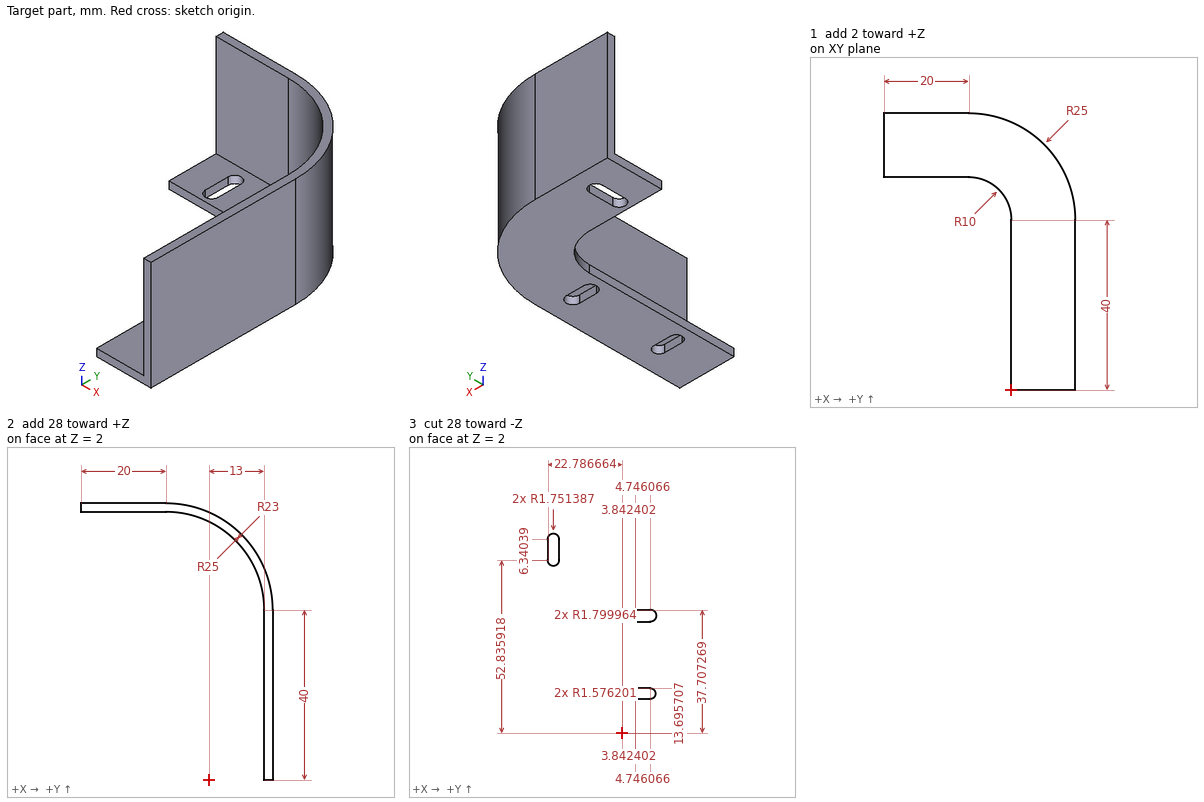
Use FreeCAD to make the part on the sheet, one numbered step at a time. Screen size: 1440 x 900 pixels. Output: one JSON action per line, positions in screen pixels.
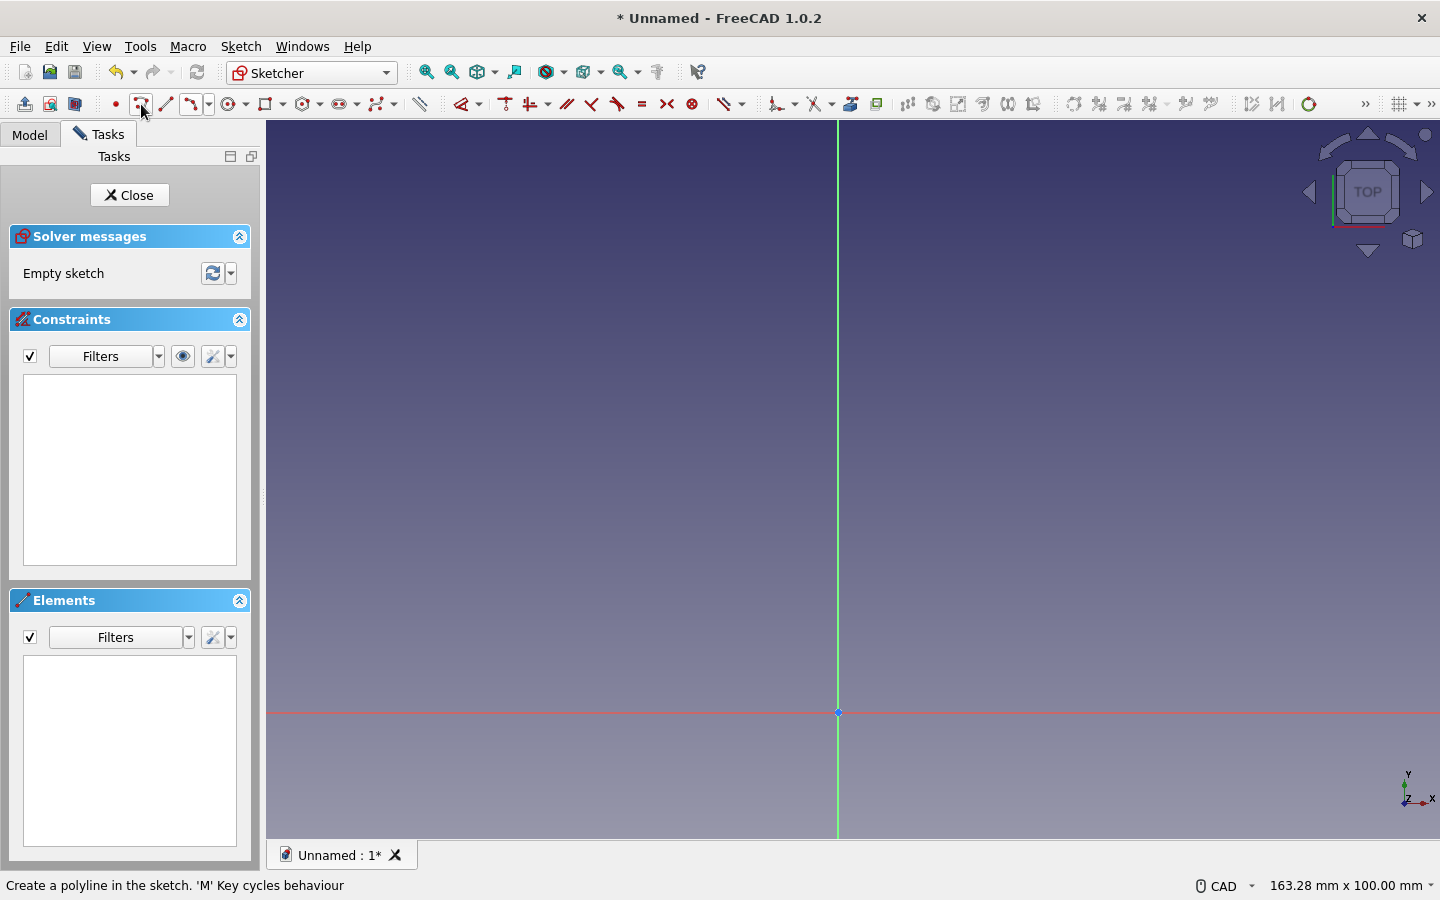
{"action": "left_click", "coordinate": [838, 425]}
{"action": "left_click", "coordinate": [838, 713]}
{"action": "left_click", "coordinate": [946, 704]}
{"action": "left_click", "coordinate": [946, 425]}
{"action": "right_click", "coordinate": [946, 425]}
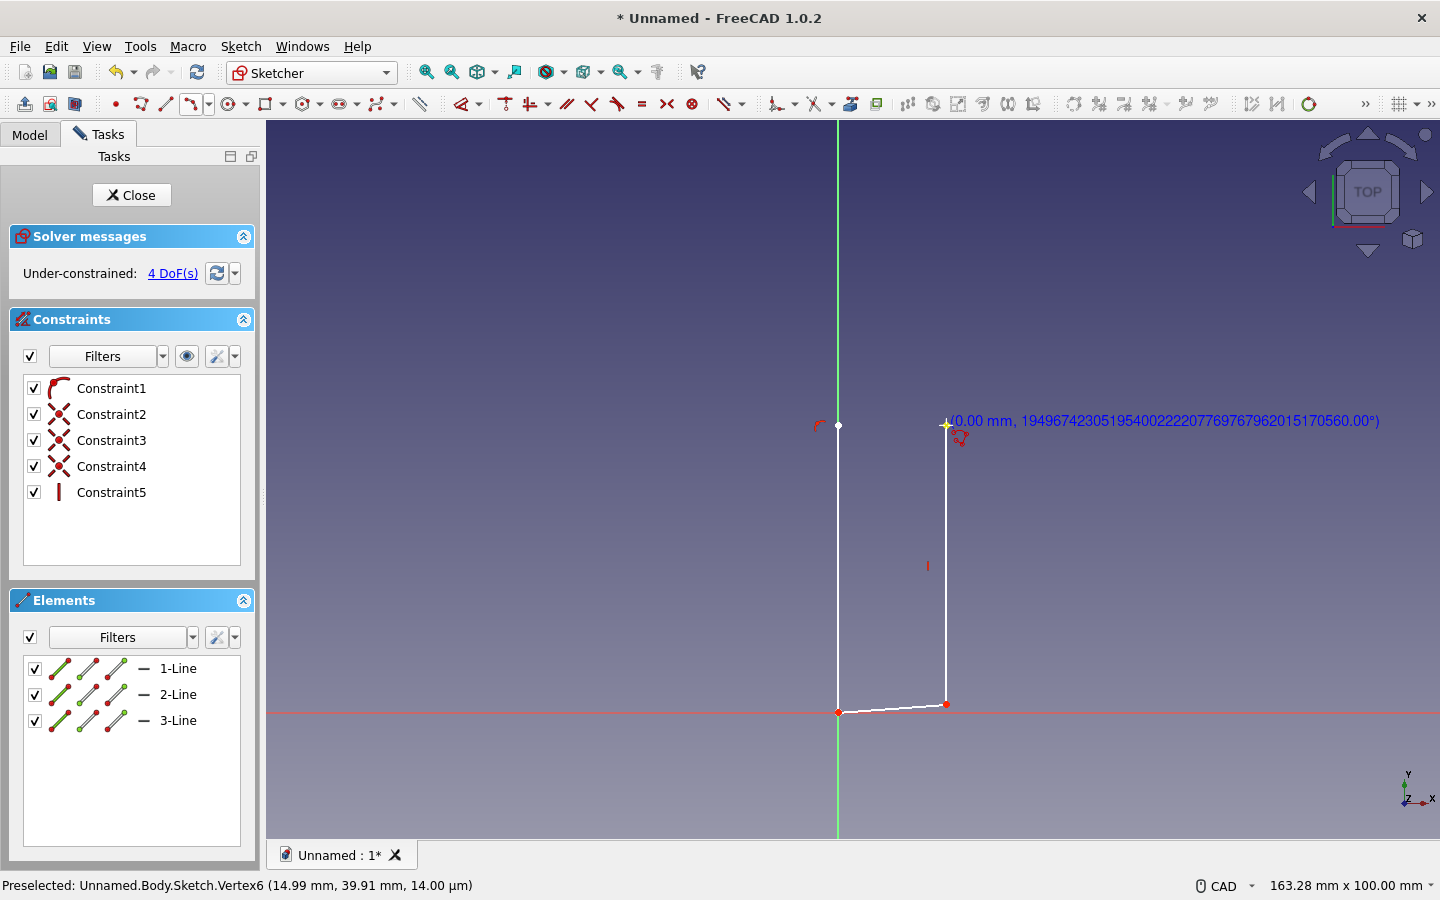
{"action": "left_click", "coordinate": [766, 246]}
{"action": "left_click", "coordinate": [623, 246]}
{"action": "left_click", "coordinate": [623, 353]}
{"action": "left_click", "coordinate": [766, 353]}
{"action": "right_click", "coordinate": [766, 353]}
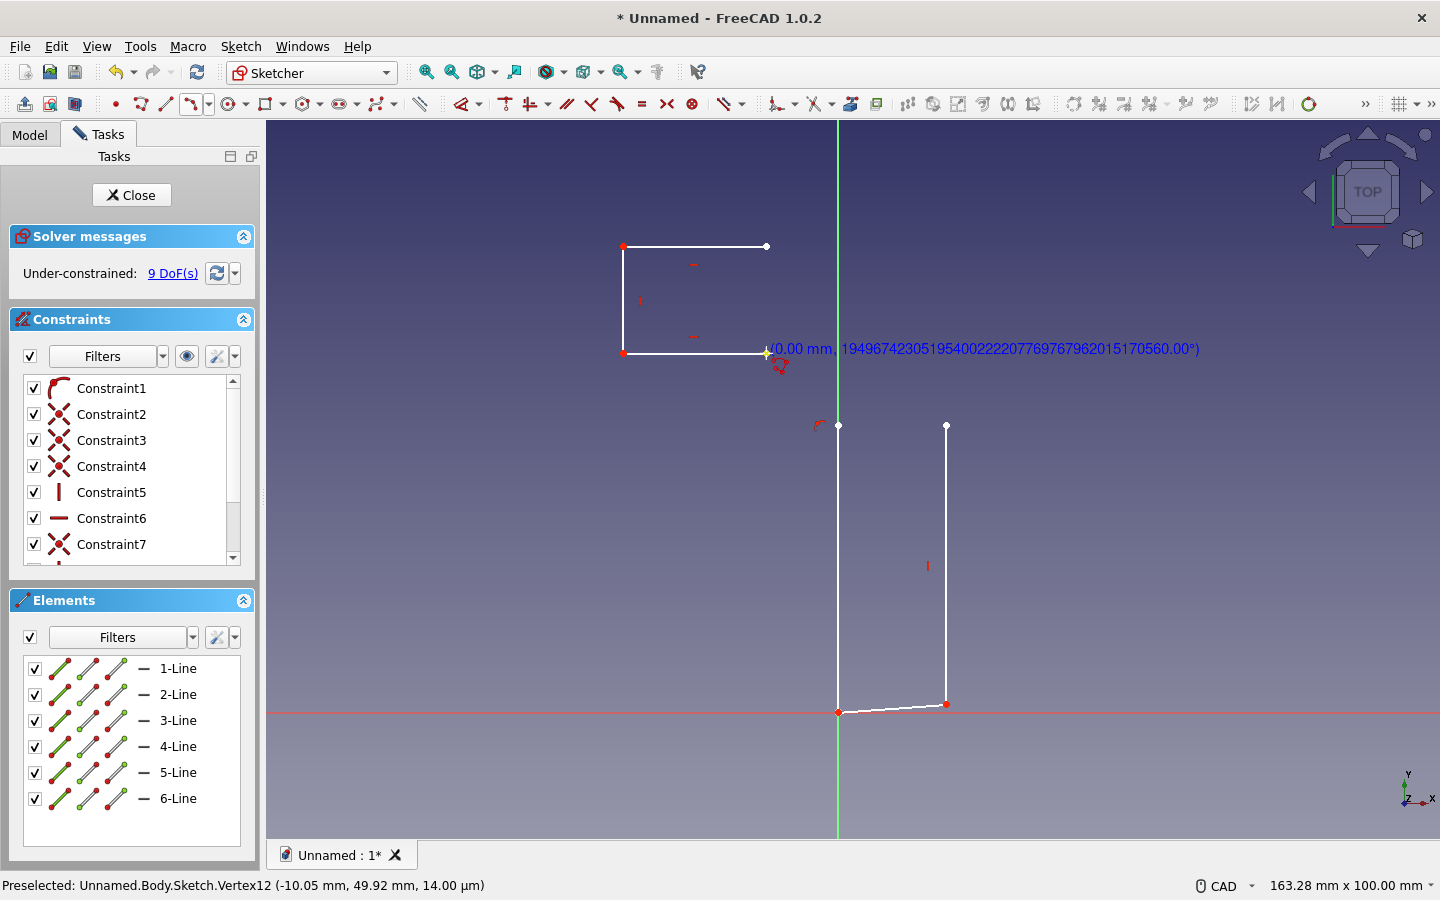
{"action": "left_click", "coordinate": [190, 104]}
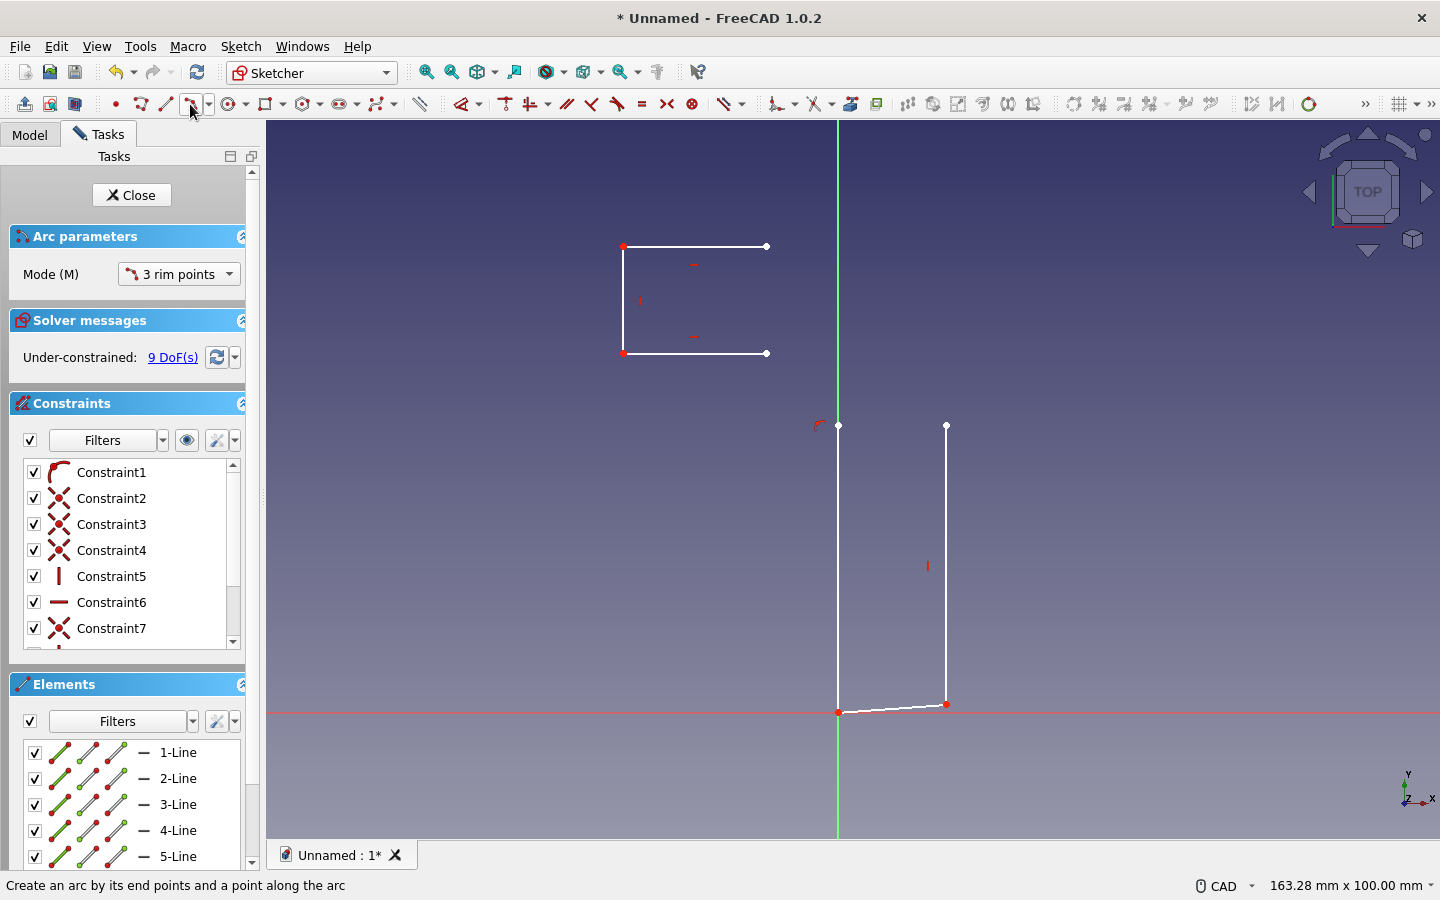
{"action": "left_click", "coordinate": [946, 426]}
{"action": "left_click", "coordinate": [766, 247]}
{"action": "left_click", "coordinate": [893, 298]}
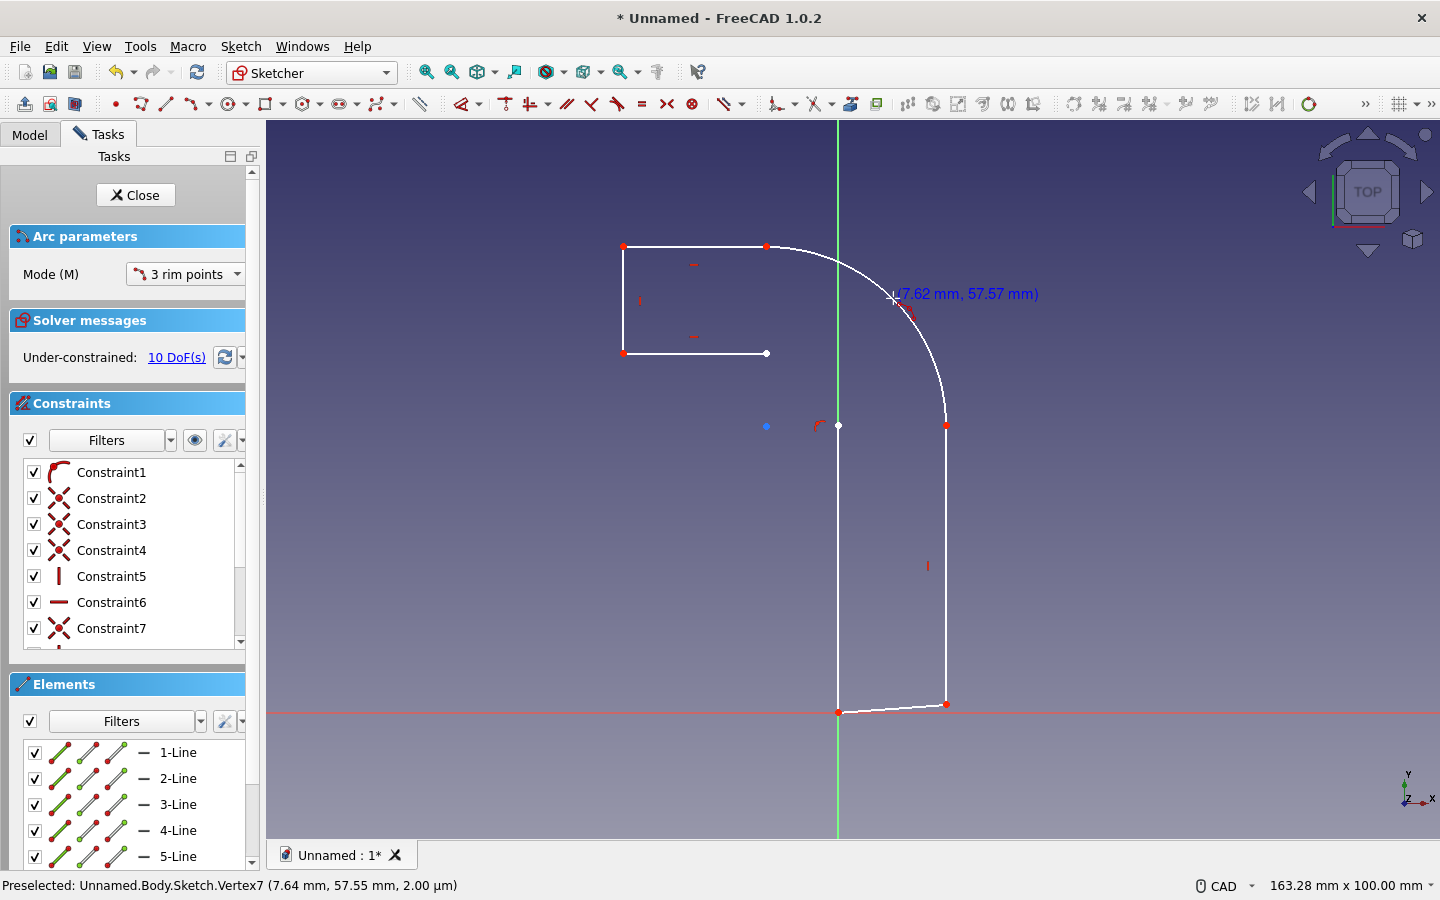
{"action": "left_click", "coordinate": [766, 354]}
{"action": "left_click", "coordinate": [838, 426]}
{"action": "left_click", "coordinate": [817, 375]}
{"action": "key", "text": "Escape"}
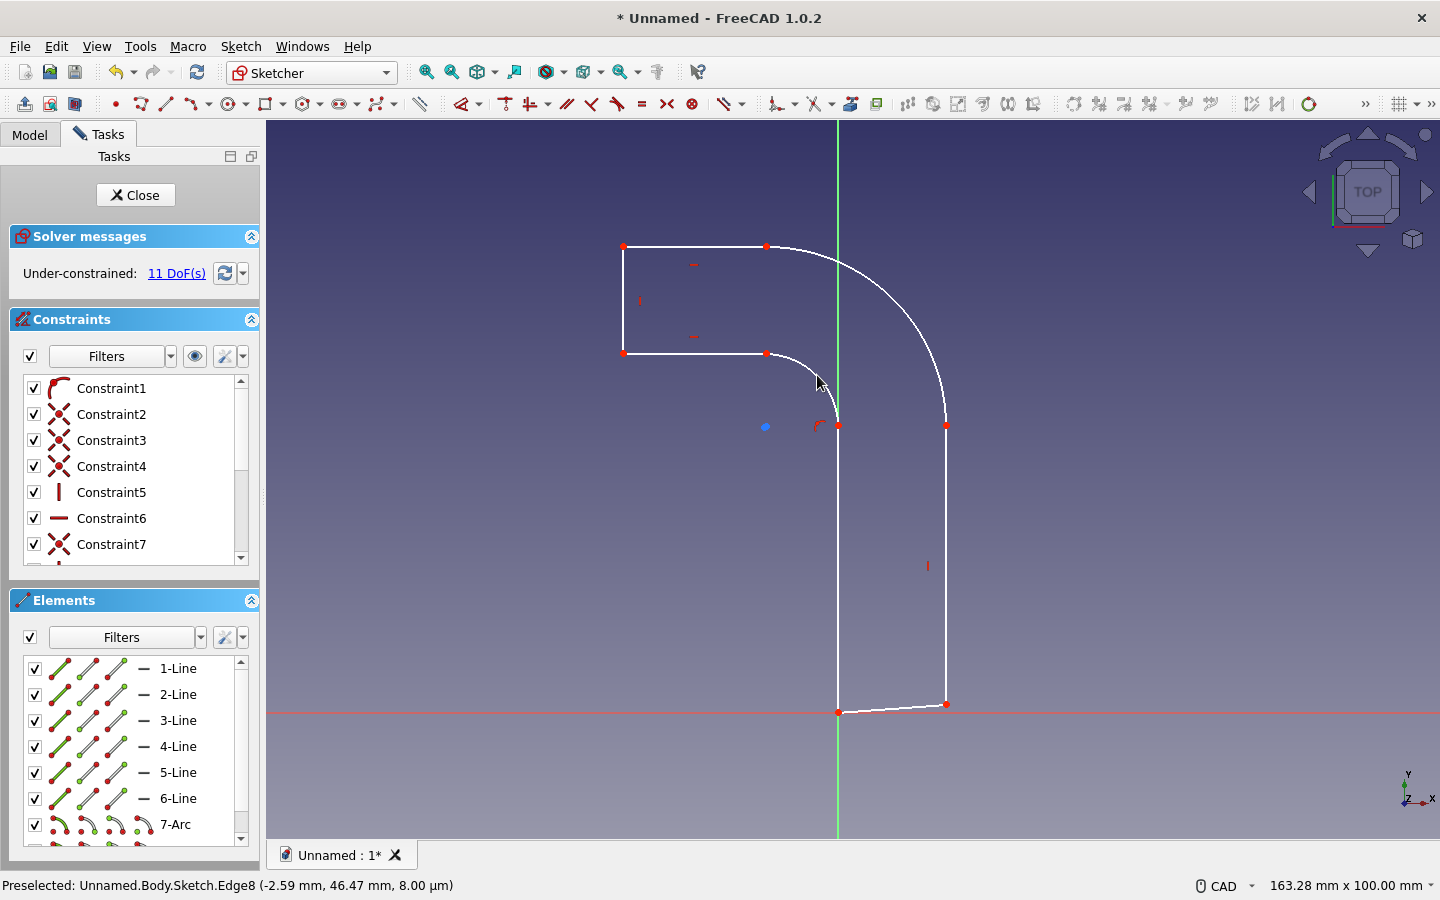
{"action": "left_click", "coordinate": [838, 512]}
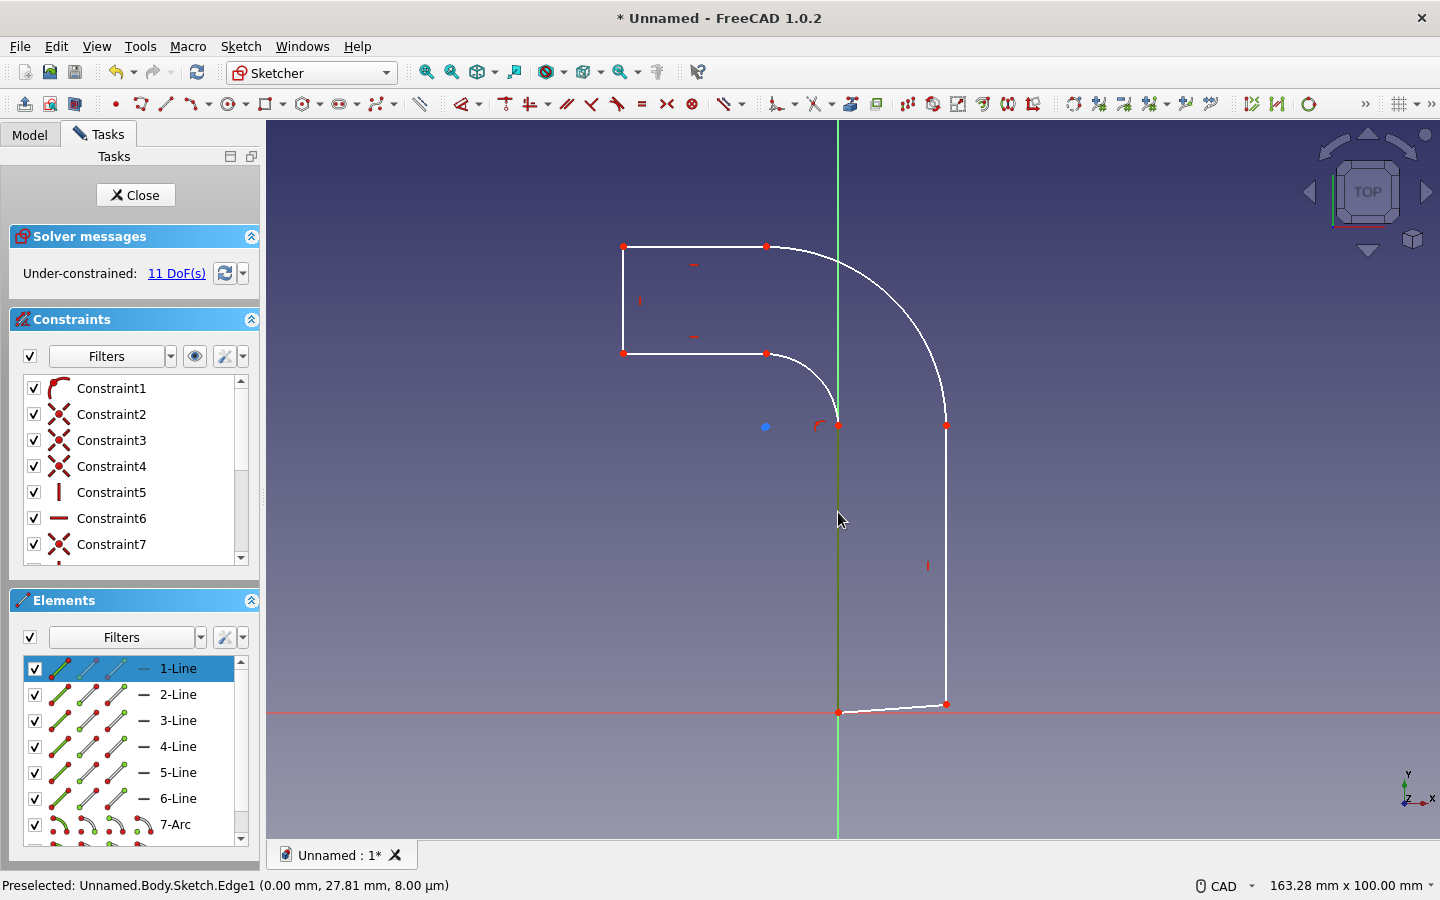
{"action": "left_click", "coordinate": [798, 362]}